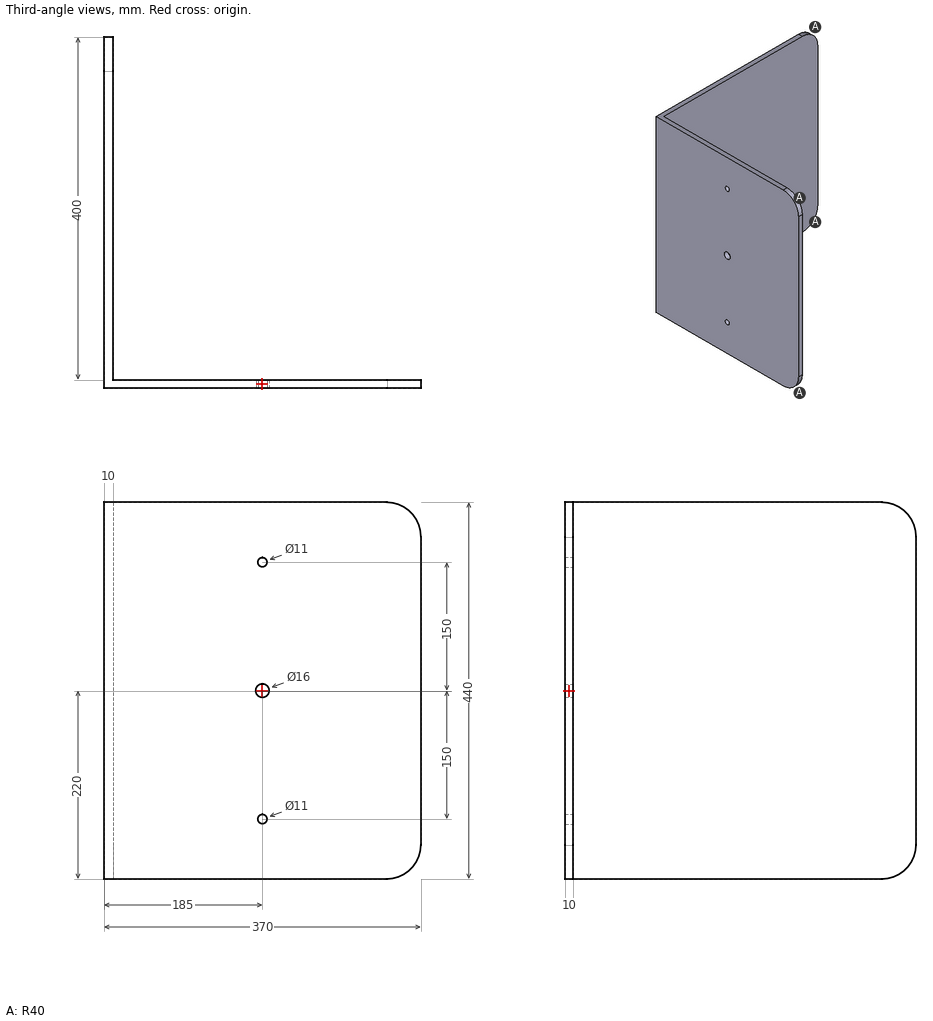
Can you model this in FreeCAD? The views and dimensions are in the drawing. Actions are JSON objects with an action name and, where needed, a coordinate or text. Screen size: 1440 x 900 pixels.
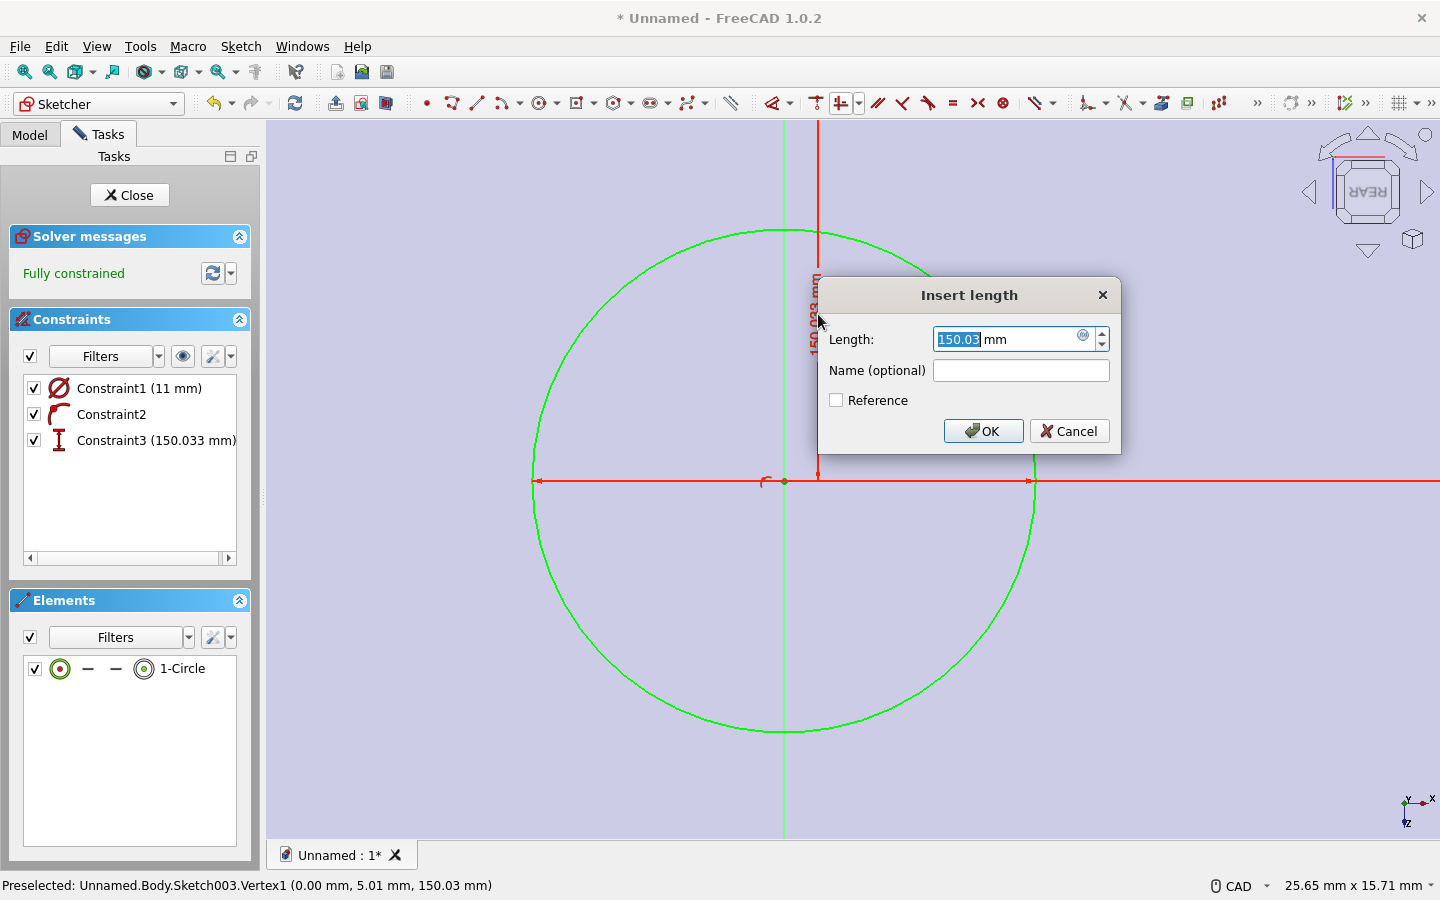
{"action": "type", "text": "150"}
{"action": "key", "text": "Return"}
{"action": "key", "text": "Escape"}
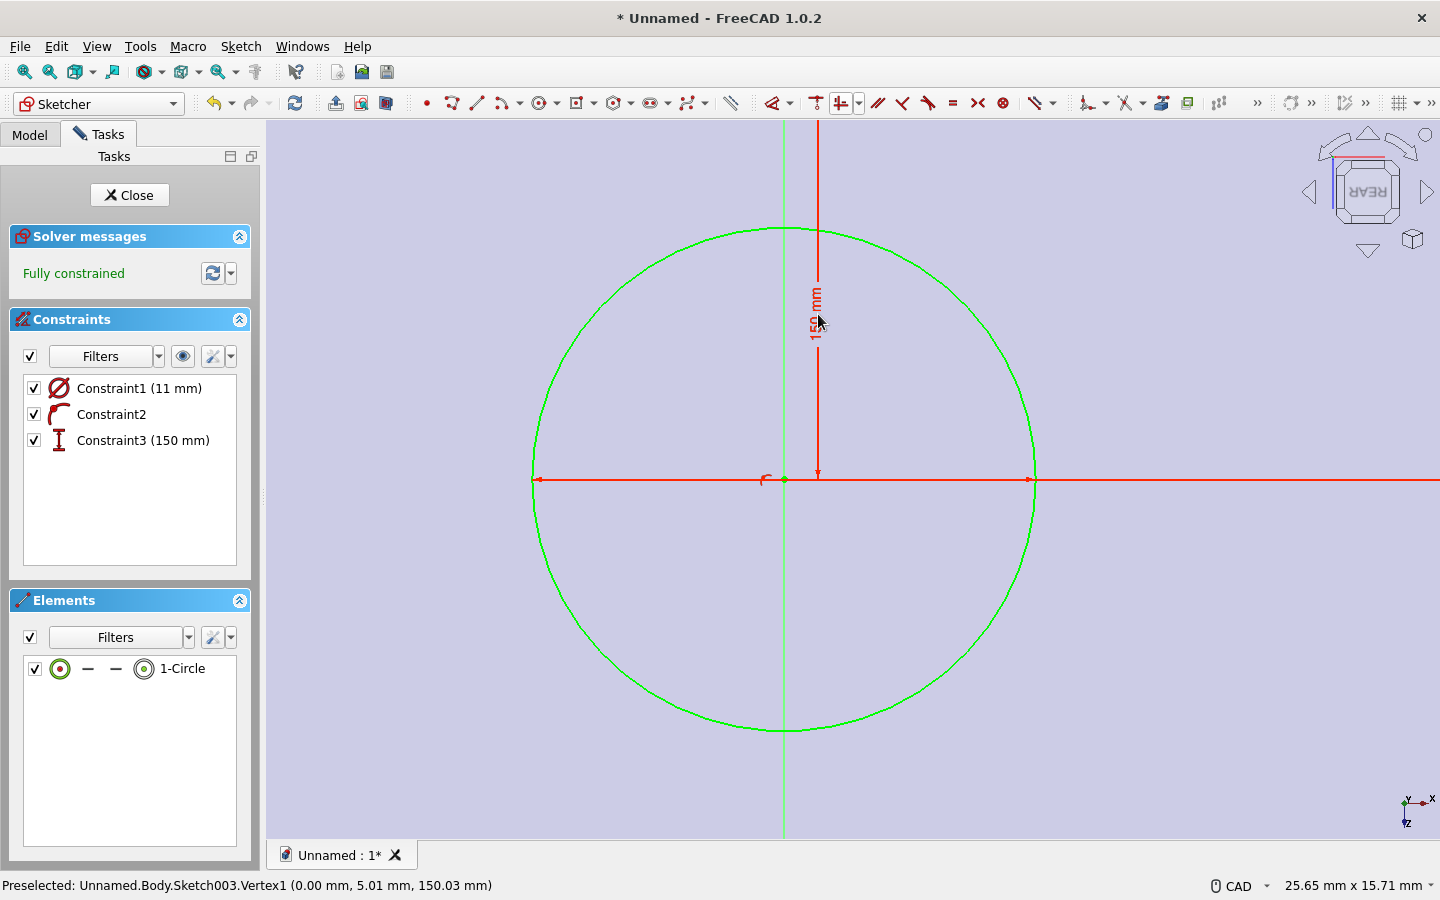
{"action": "left_click", "coordinate": [130, 195]}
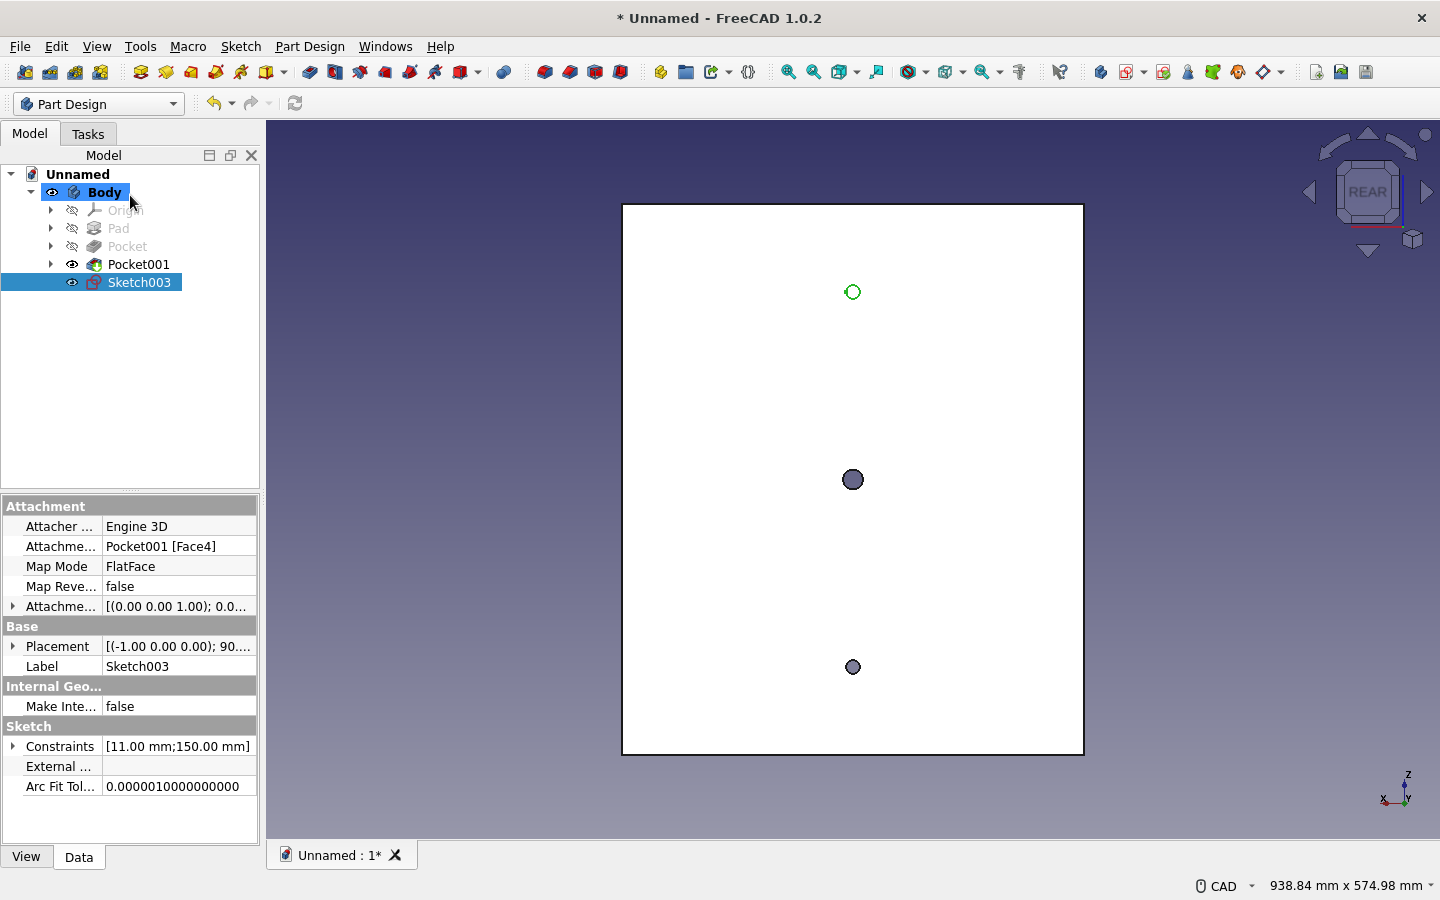
{"action": "left_click", "coordinate": [310, 72]}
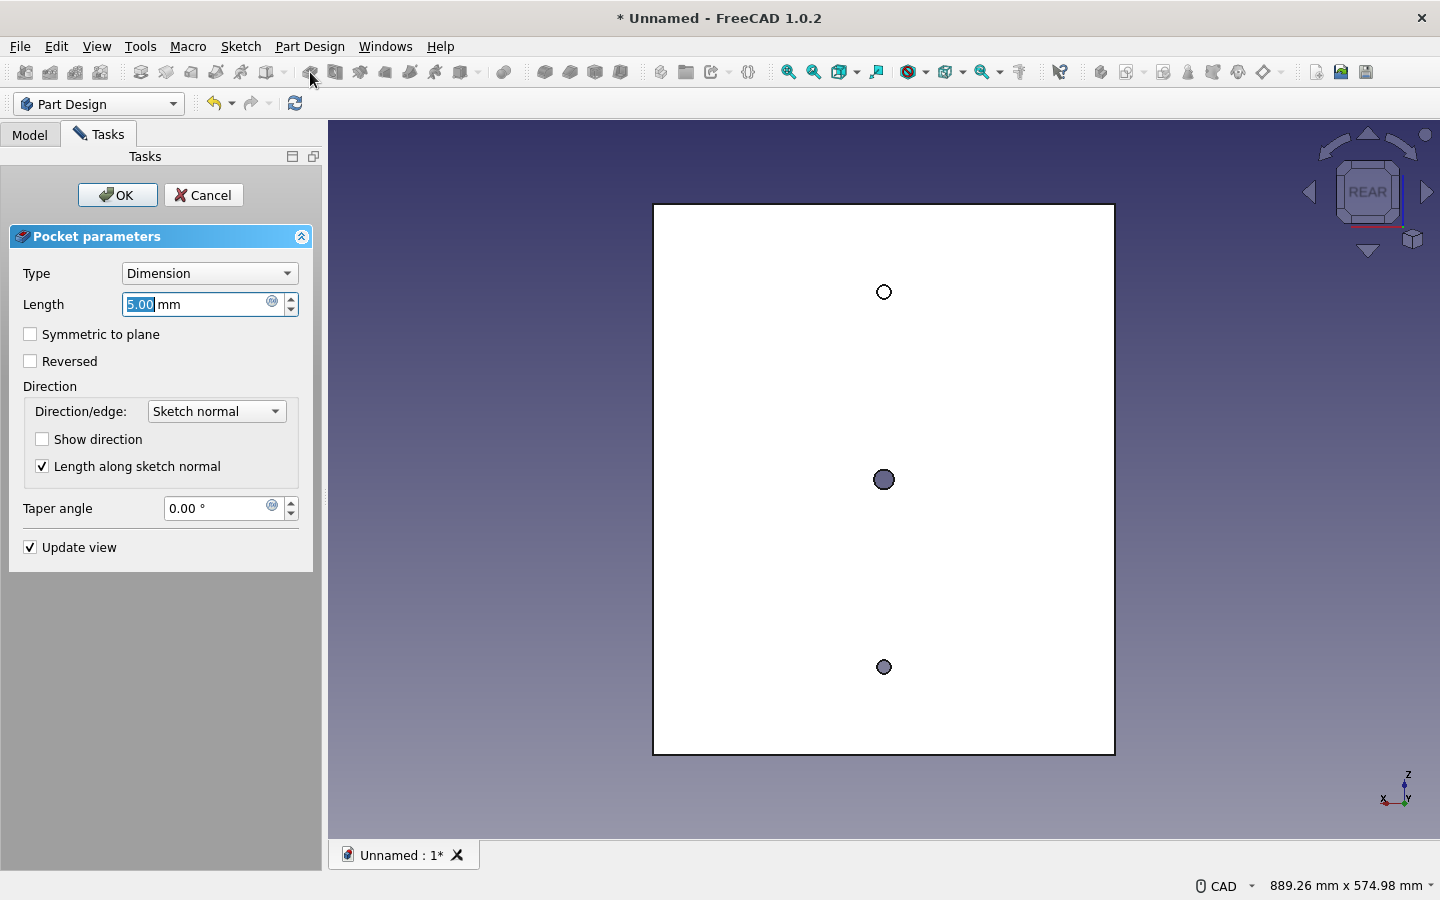
{"action": "left_click", "coordinate": [210, 274]}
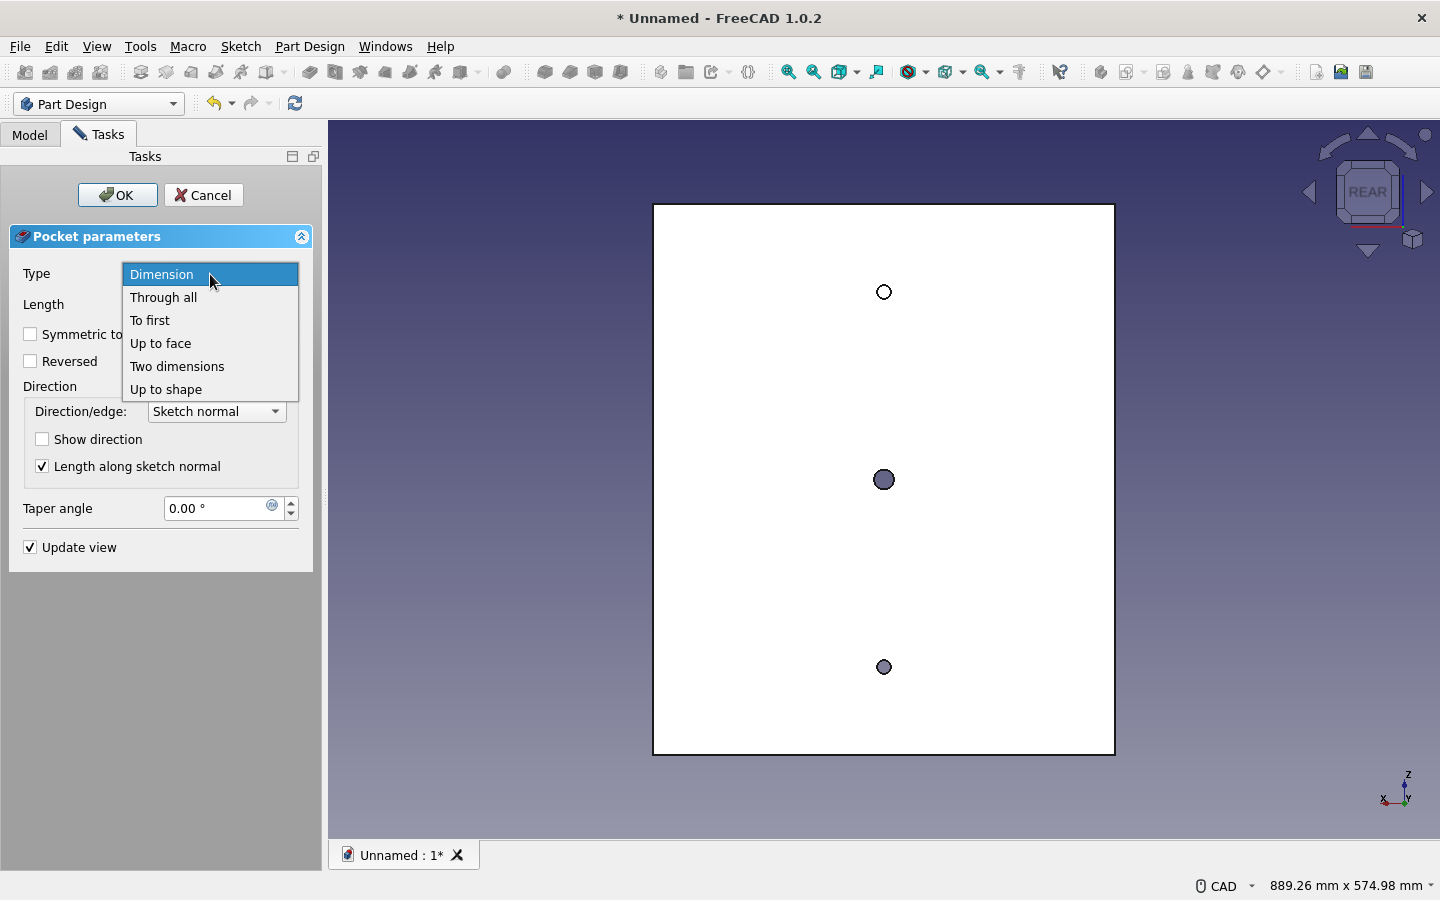
{"action": "left_click", "coordinate": [208, 320]}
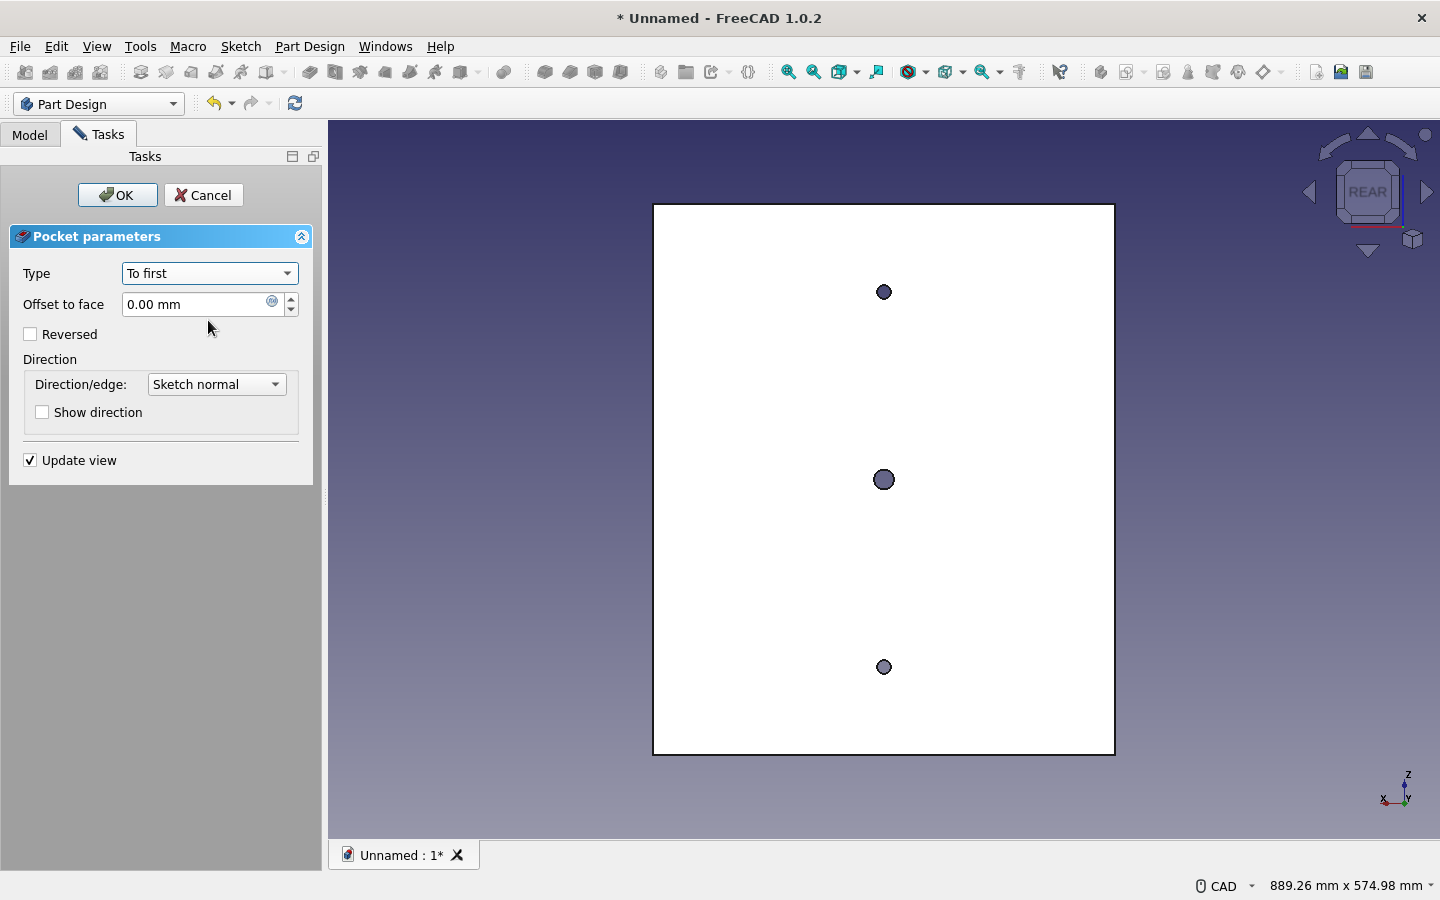
{"action": "left_click", "coordinate": [118, 195]}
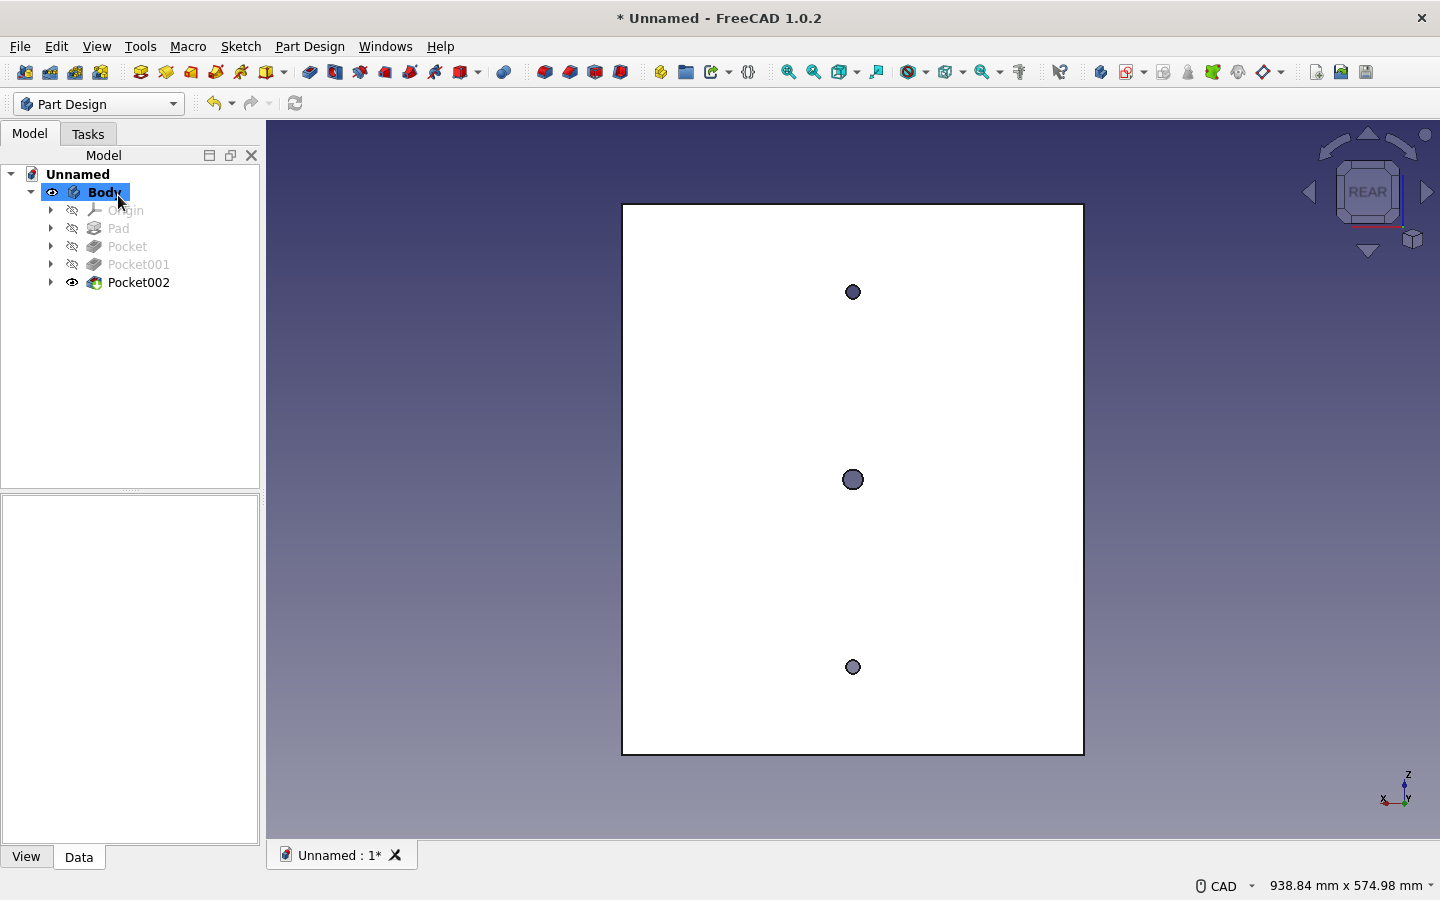
{"action": "left_click", "coordinate": [985, 321]}